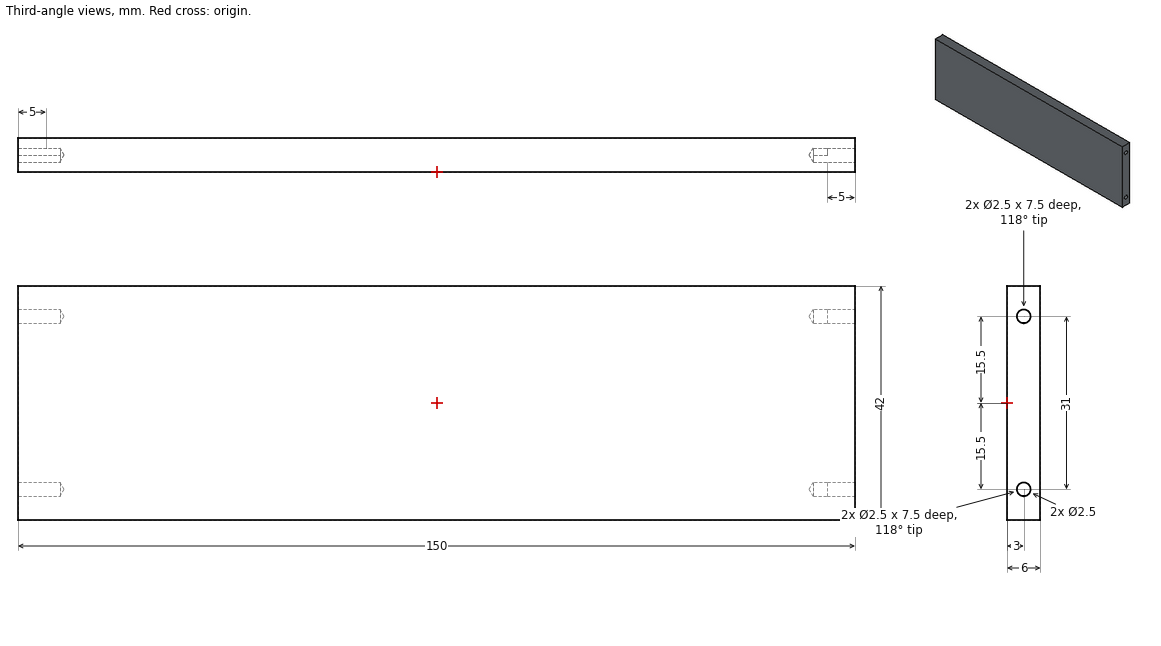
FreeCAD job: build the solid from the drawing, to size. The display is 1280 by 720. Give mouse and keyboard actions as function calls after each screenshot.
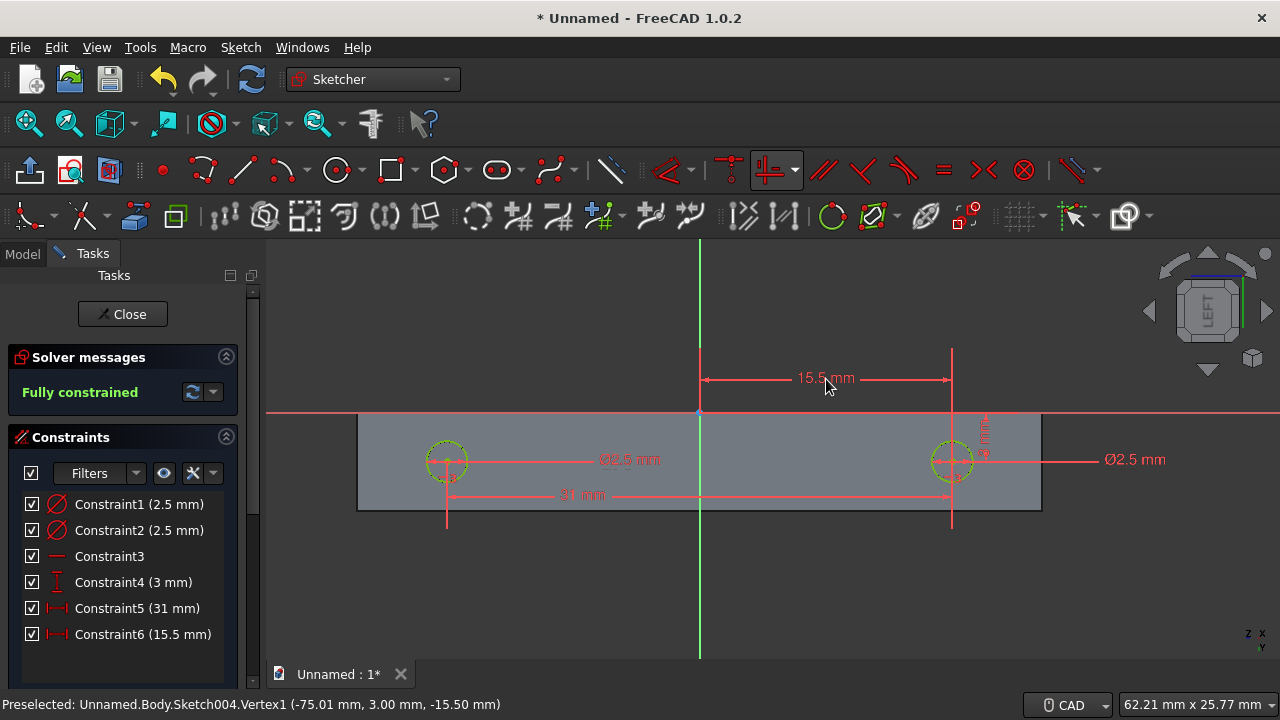
click(123, 314)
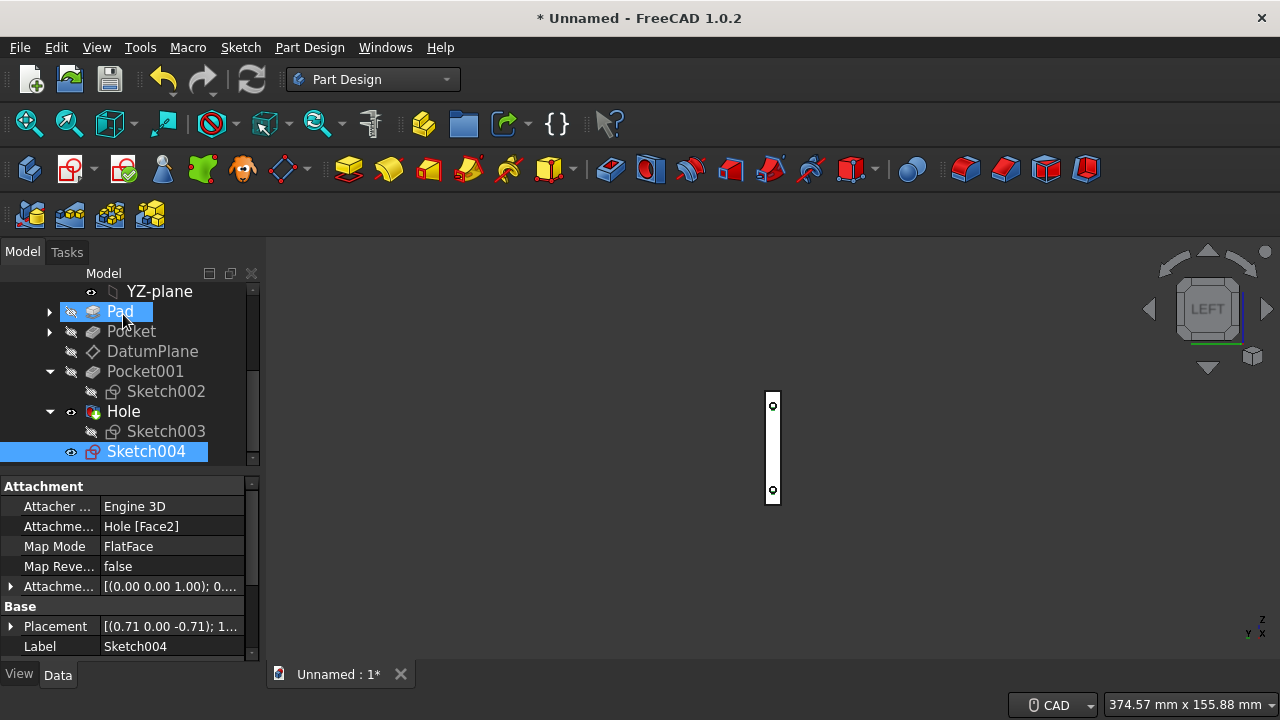
click(652, 170)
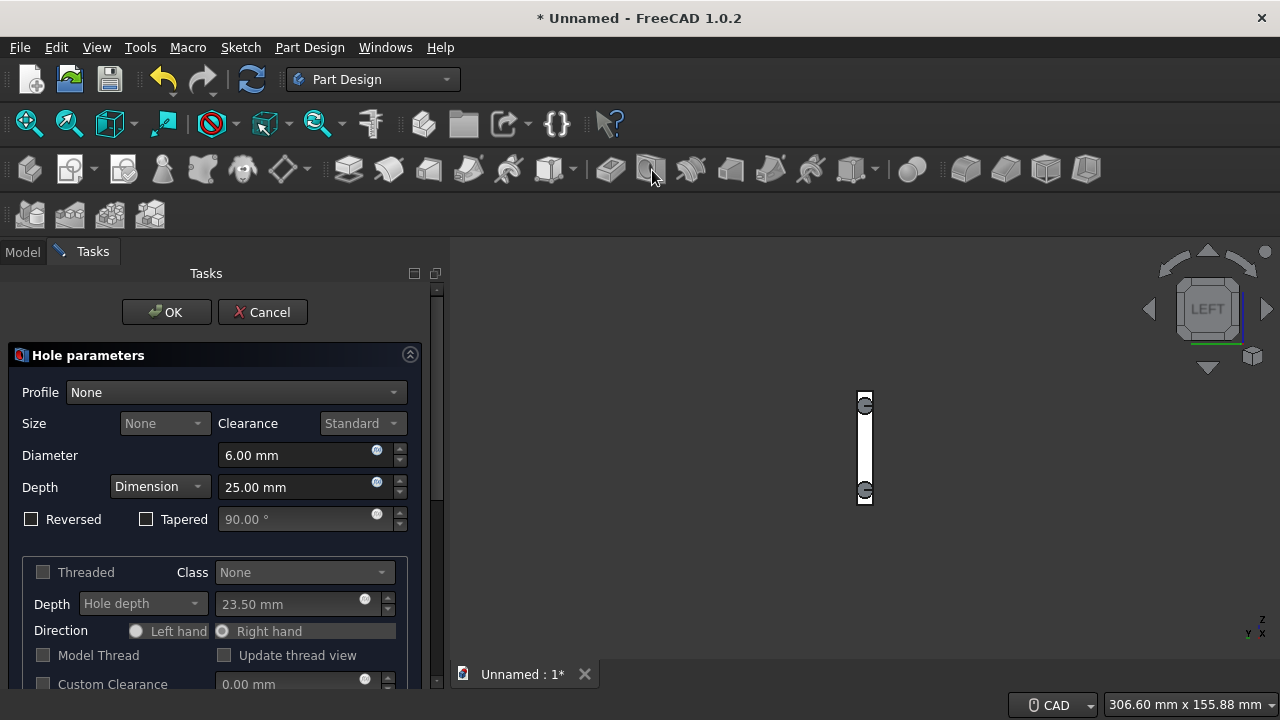
triple_click(305, 455)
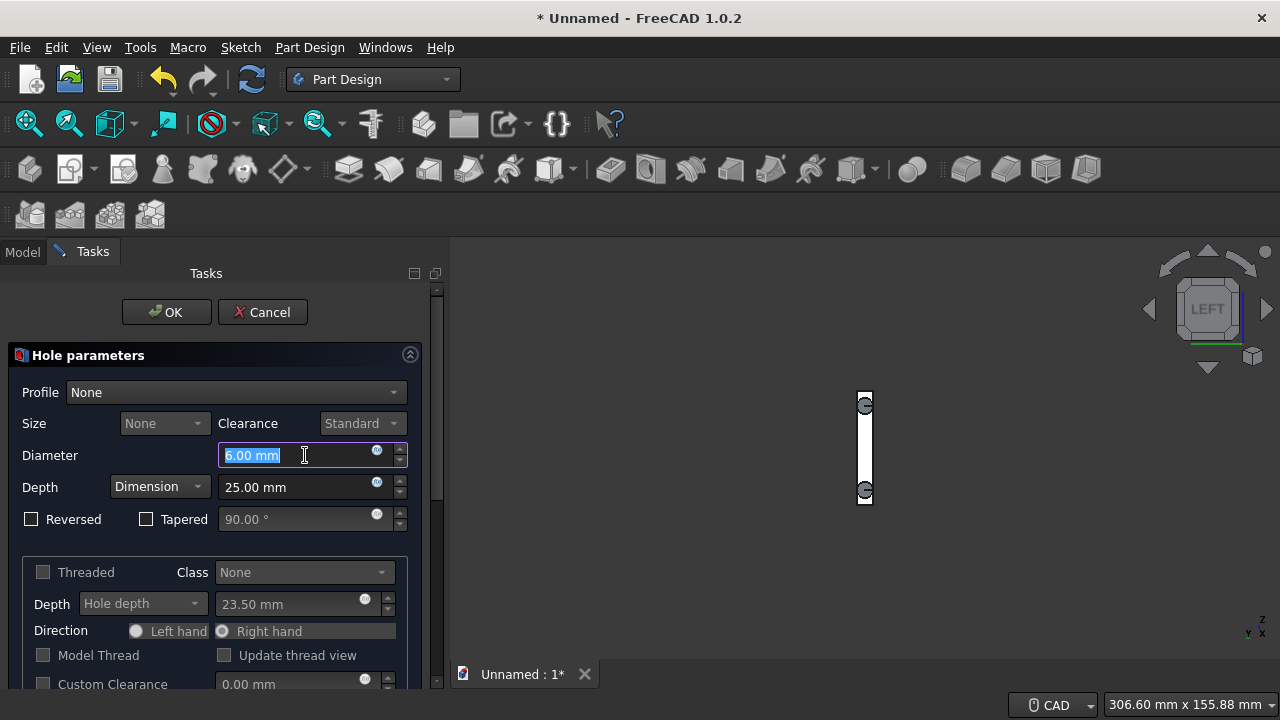
text(2.5)
key(Tab)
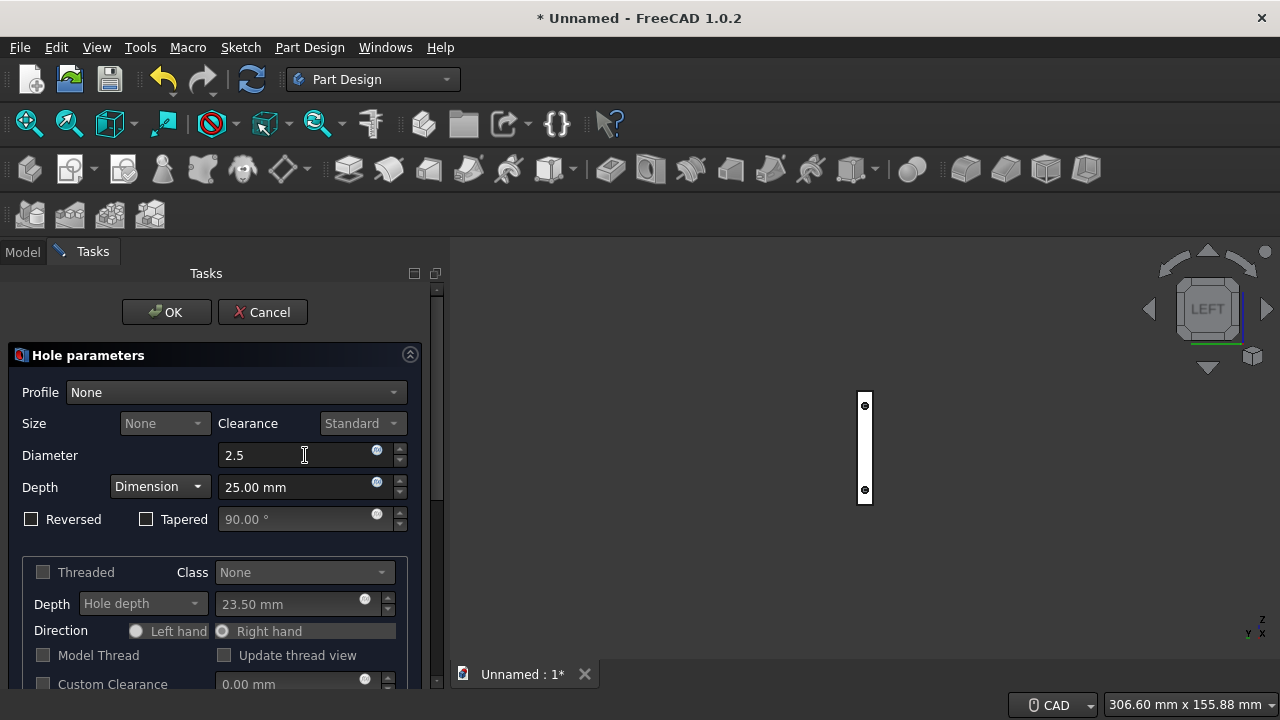
triple_click(305, 487)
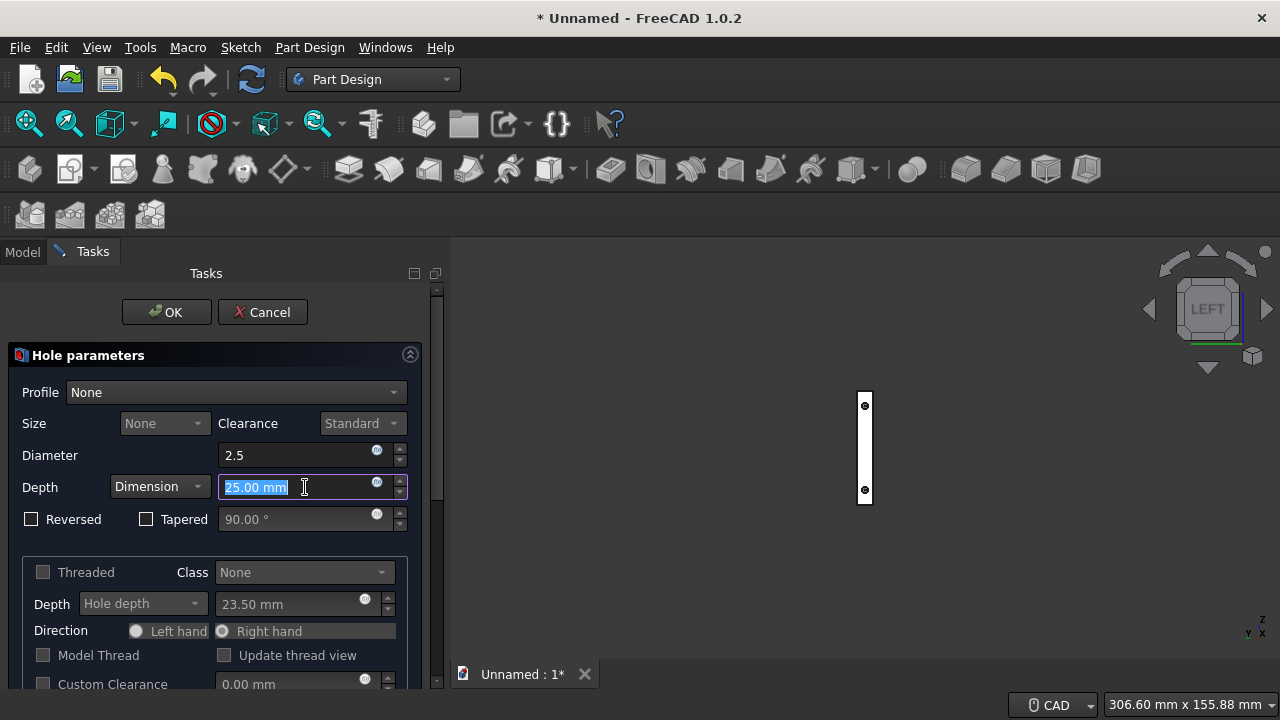
text(7.5)
key(Tab)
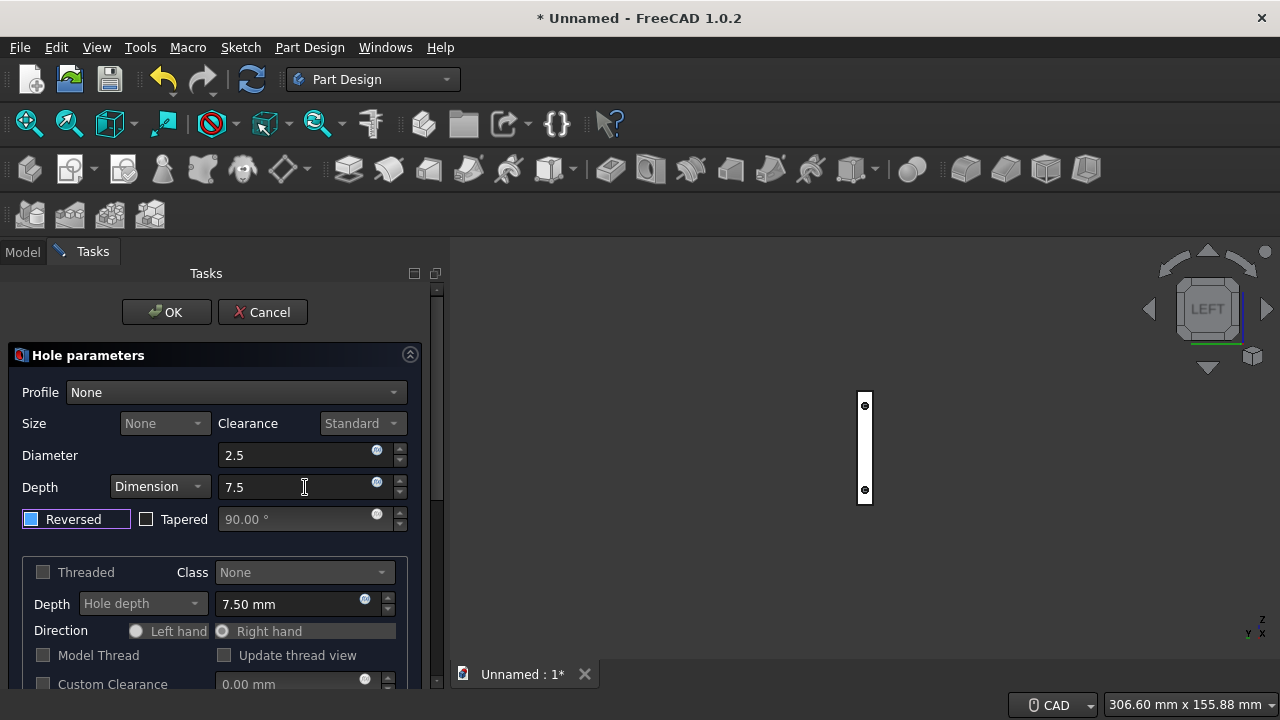
click(167, 312)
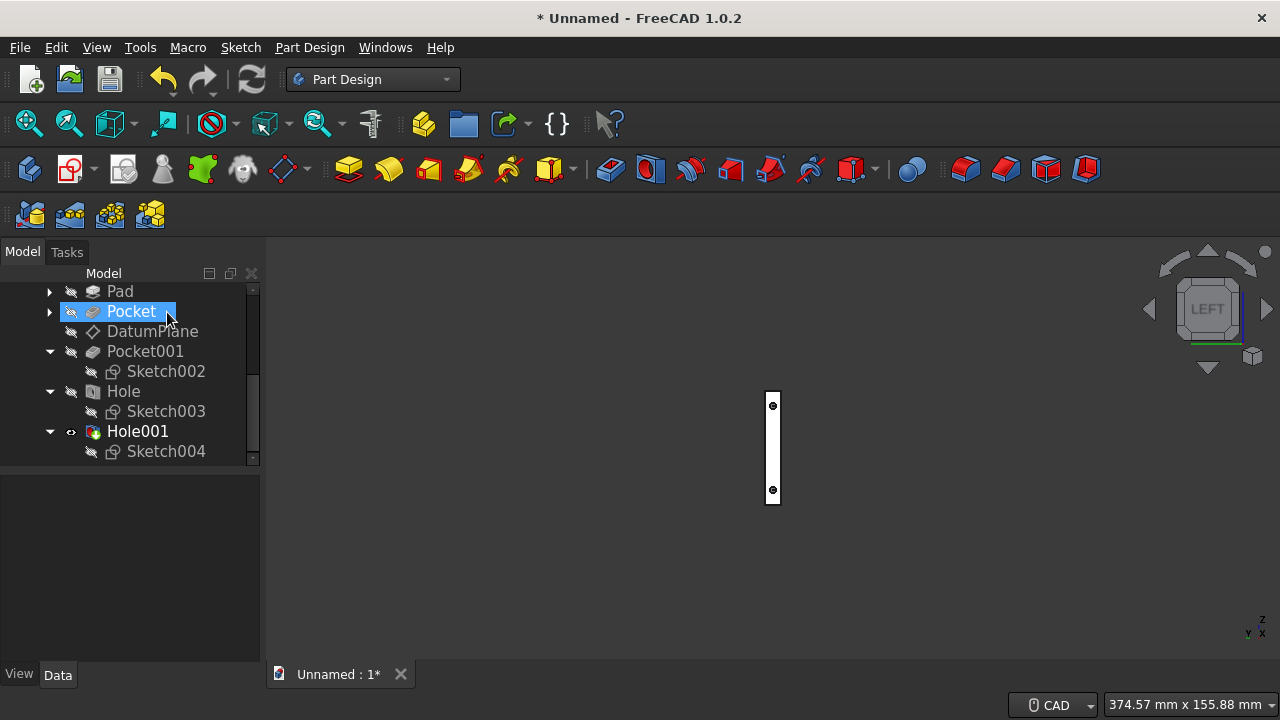
key(0)